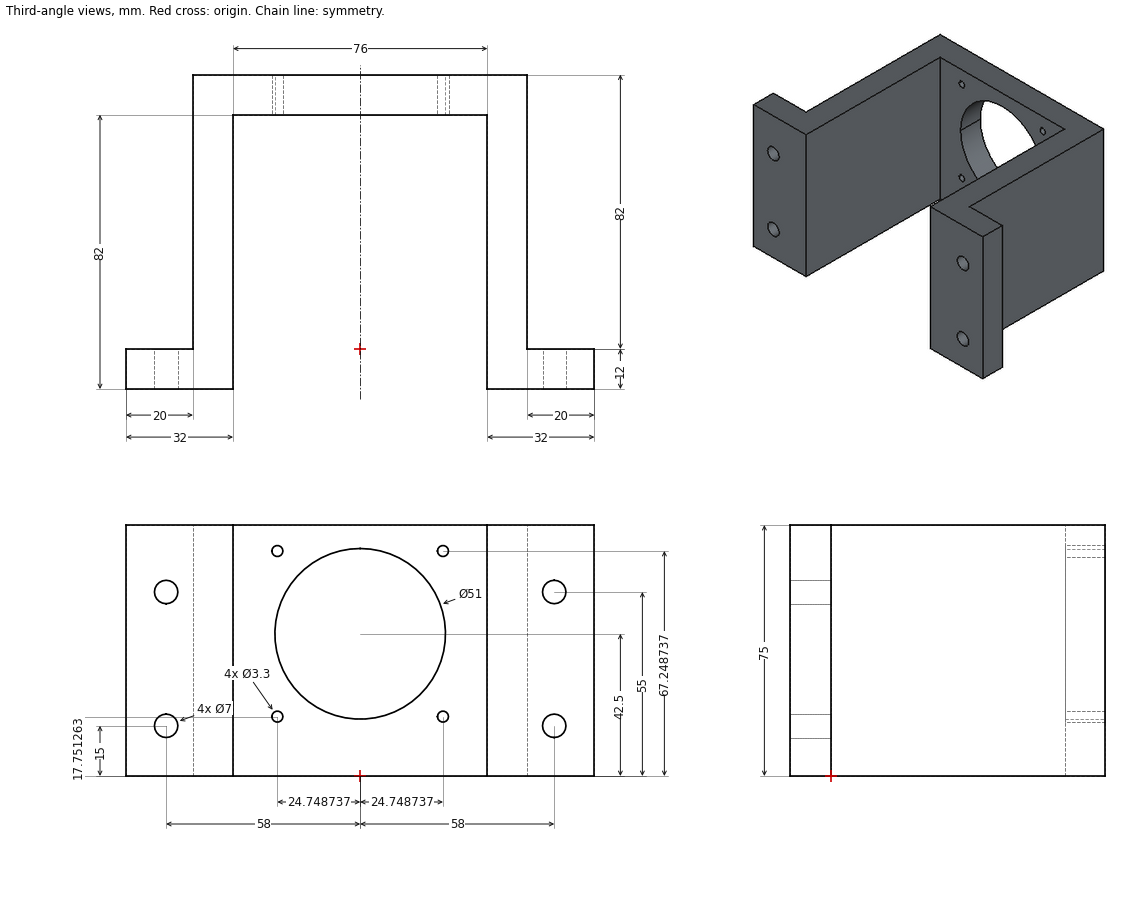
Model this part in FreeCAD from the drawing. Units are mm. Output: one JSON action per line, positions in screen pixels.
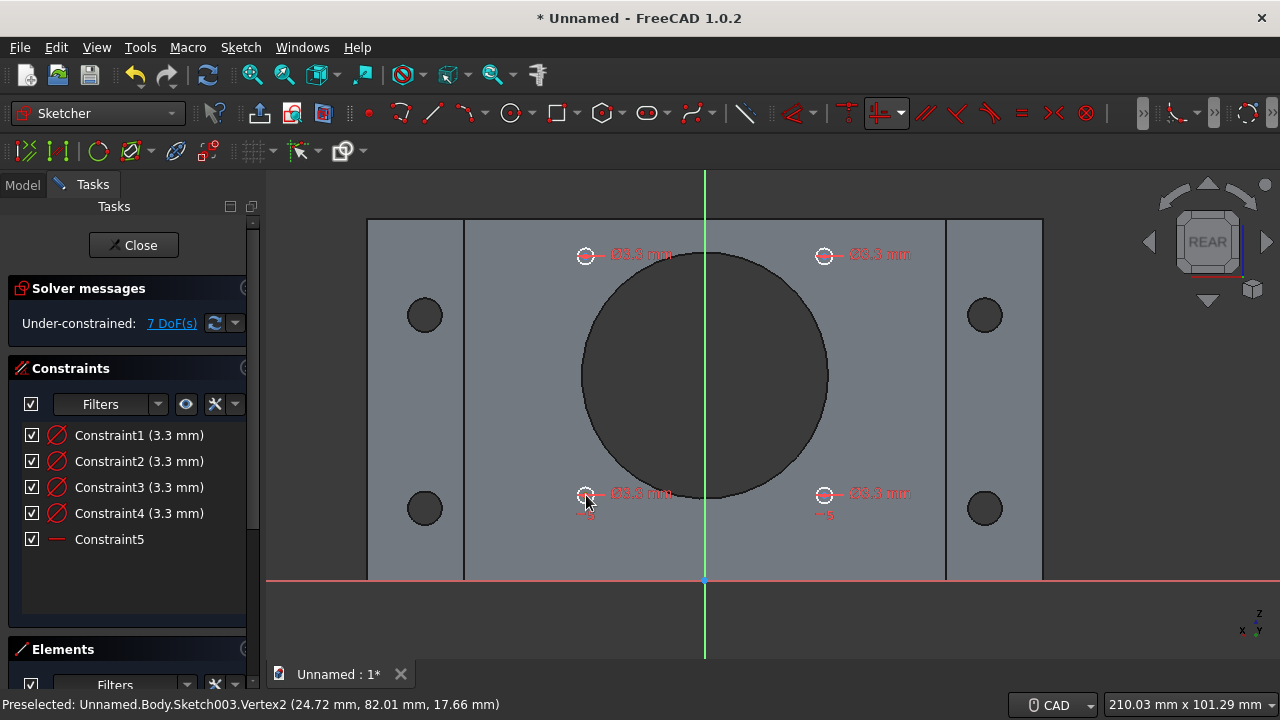
{"action": "left_click", "coordinate": [586, 256]}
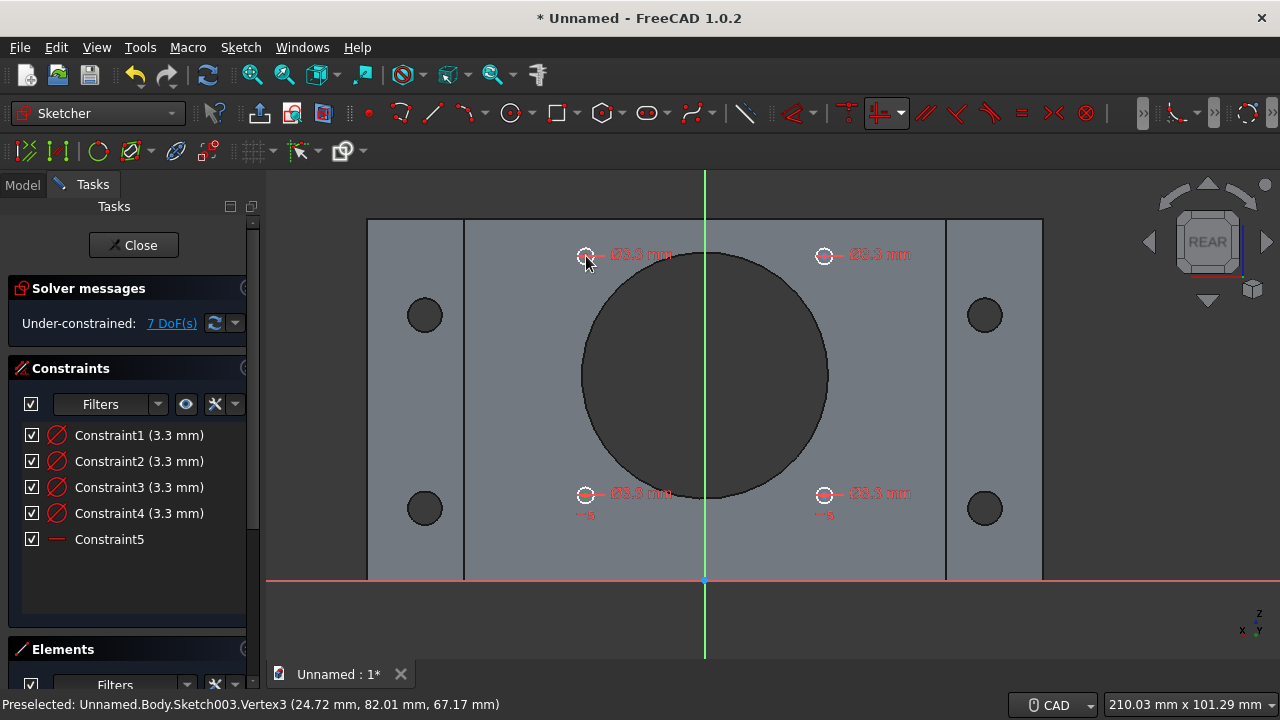
{"action": "left_click", "coordinate": [904, 114]}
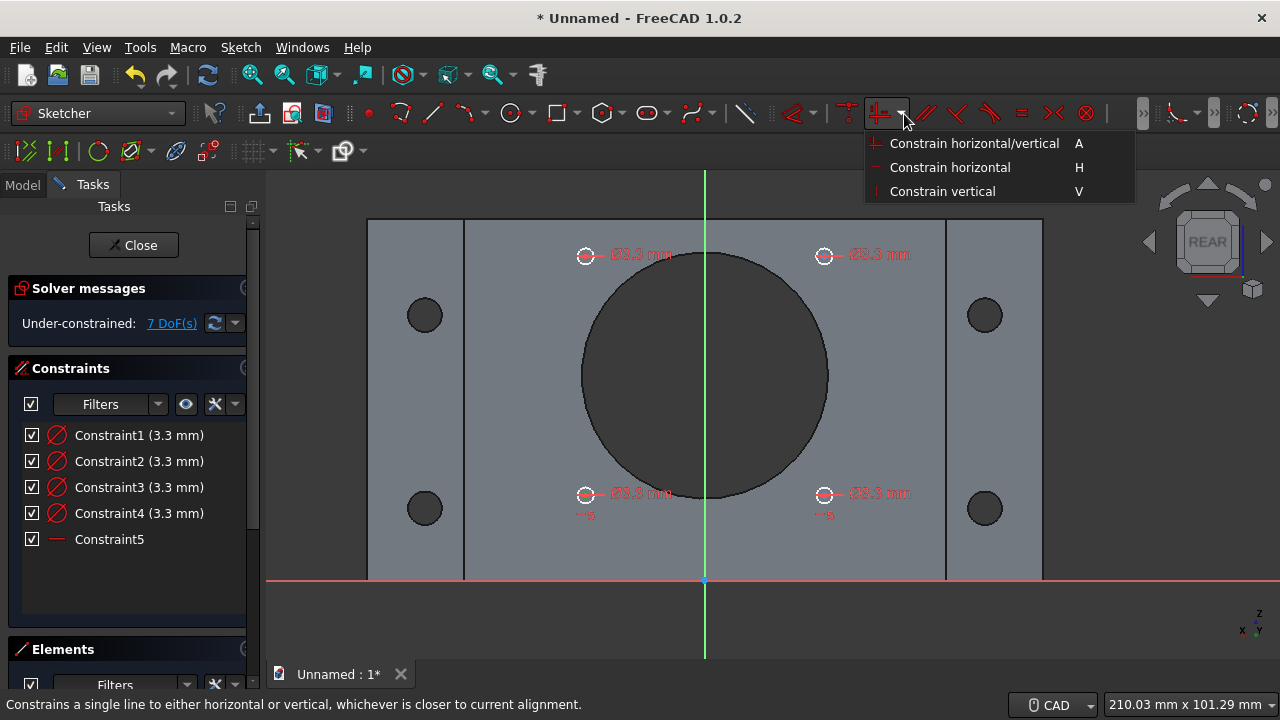
{"action": "left_click", "coordinate": [1000, 191]}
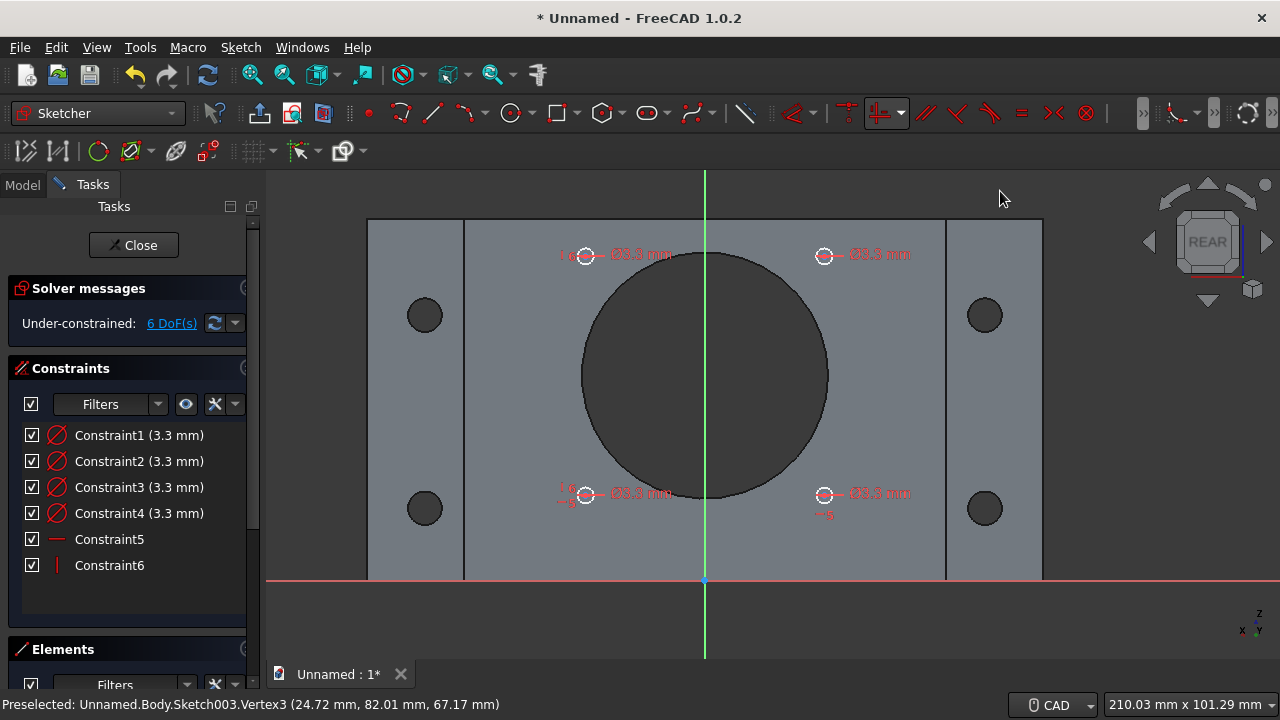
{"action": "left_click", "coordinate": [824, 495]}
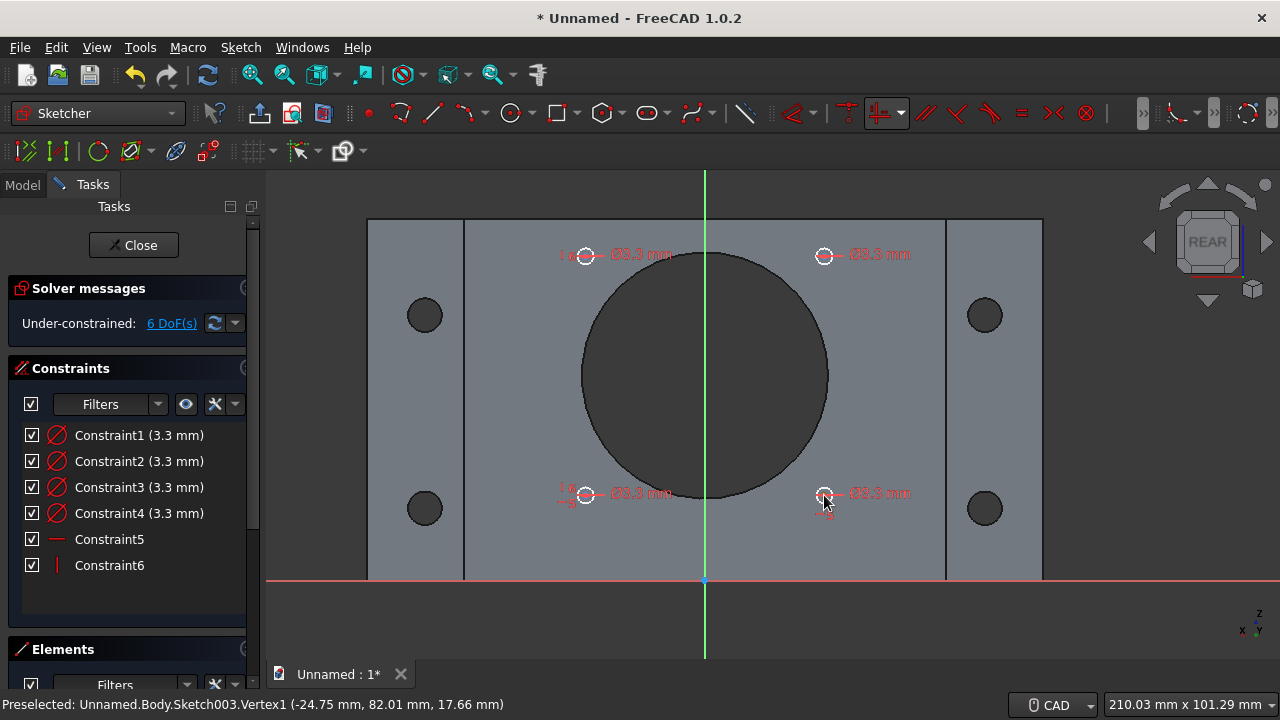
{"action": "left_click", "coordinate": [824, 256]}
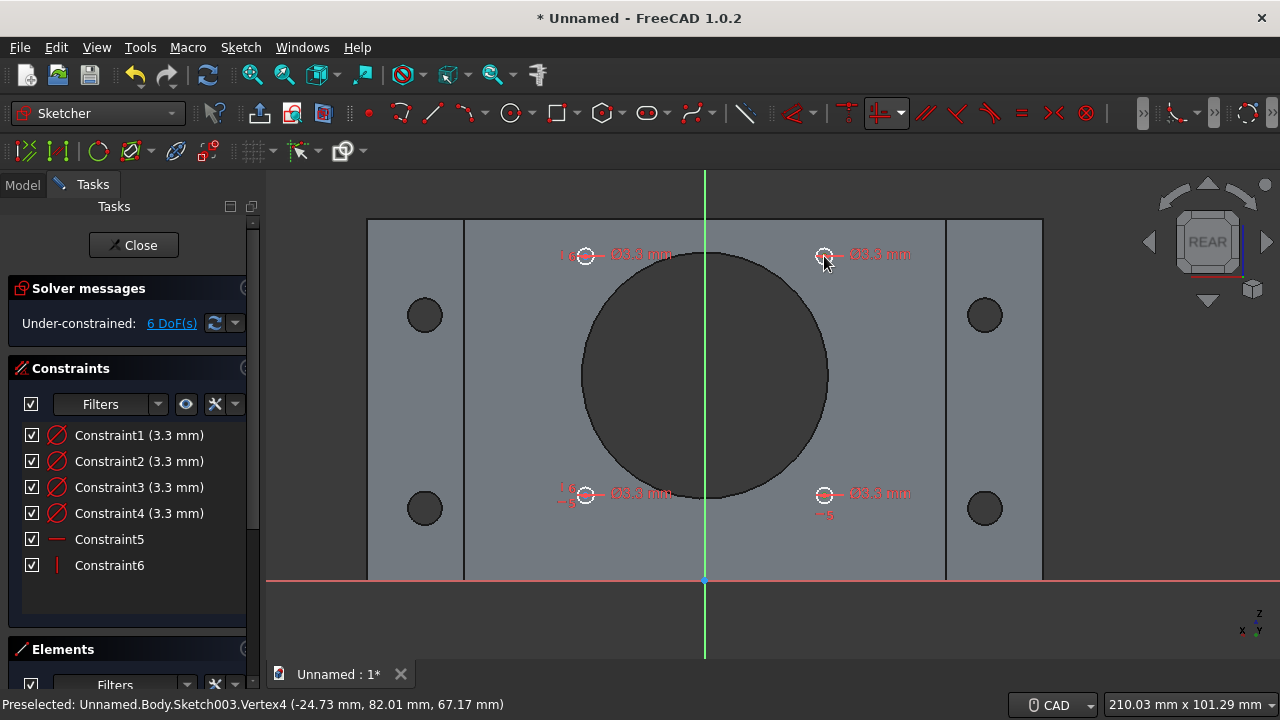
{"action": "key", "text": "v"}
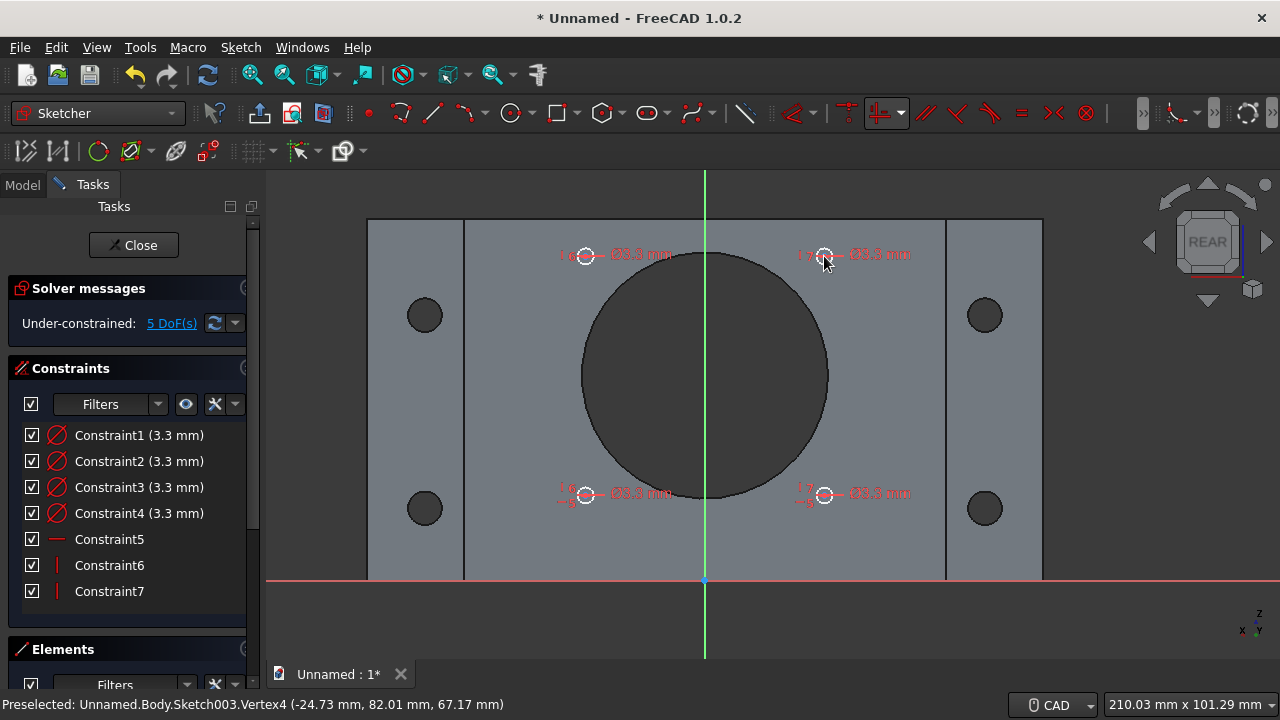
{"action": "left_click", "coordinate": [586, 256]}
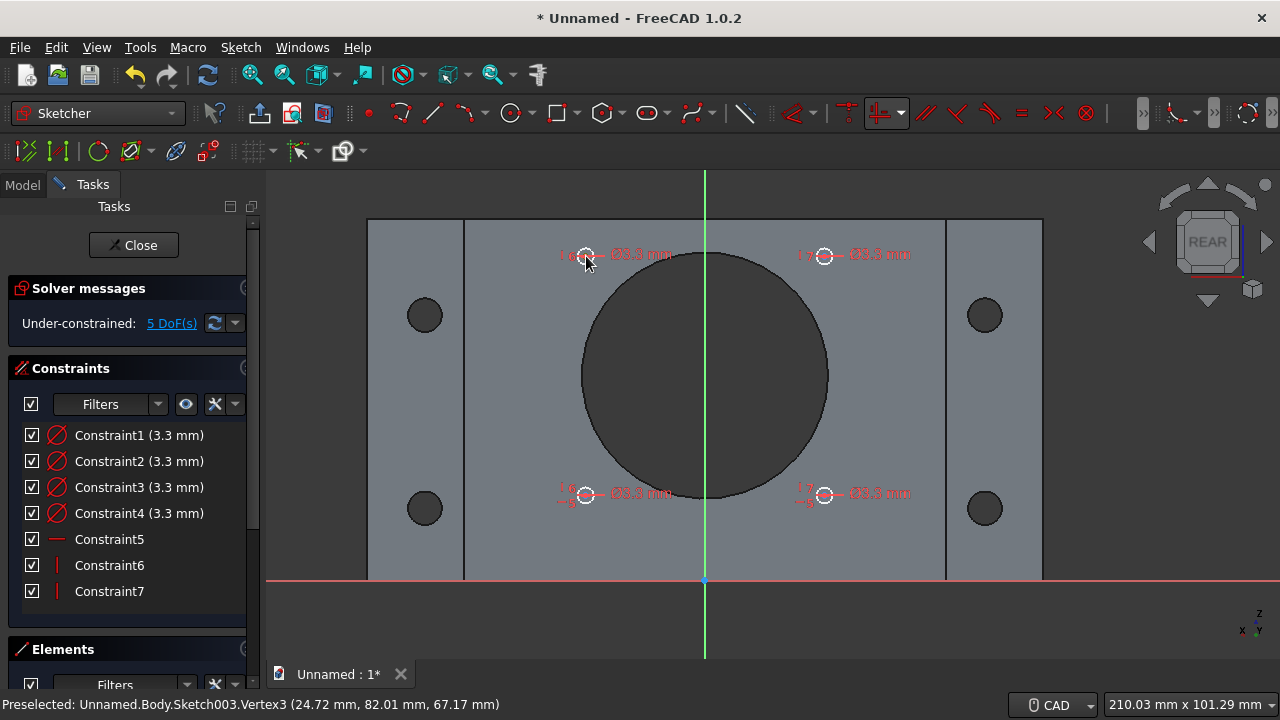
{"action": "left_click", "coordinate": [824, 256]}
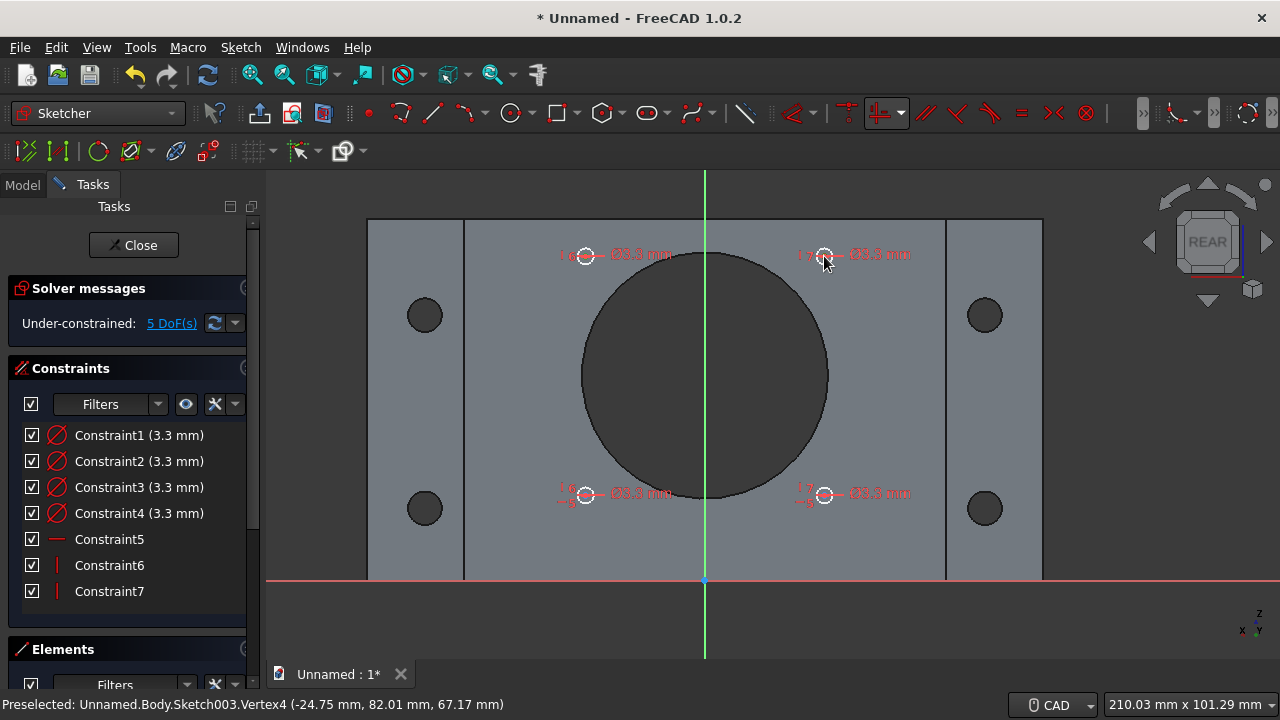
{"action": "left_click", "coordinate": [904, 114]}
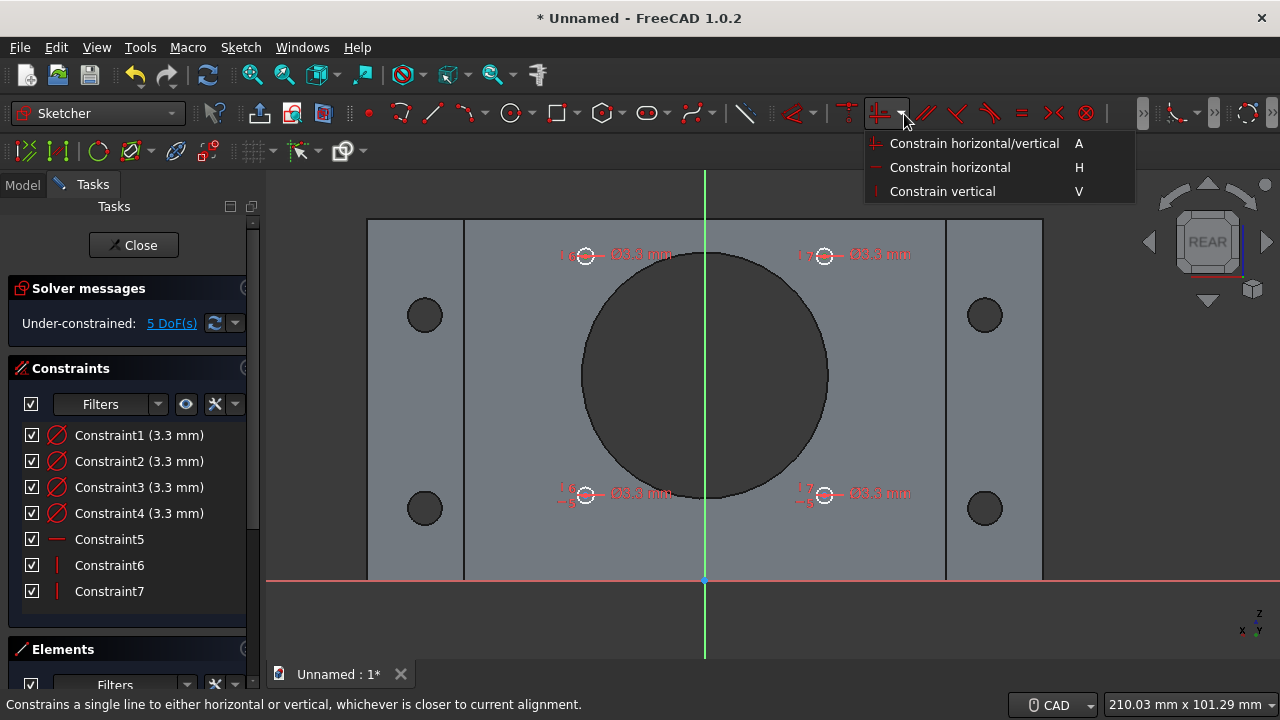
{"action": "left_click", "coordinate": [1000, 167]}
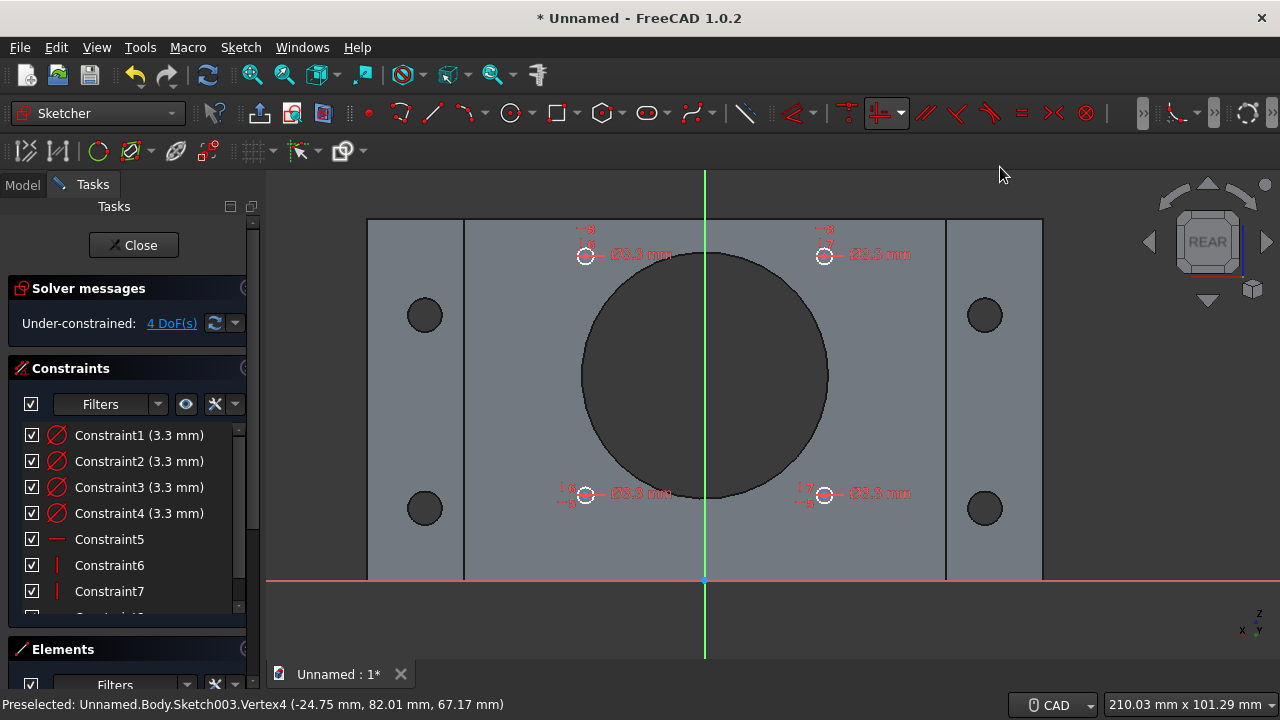
{"action": "left_click", "coordinate": [792, 114]}